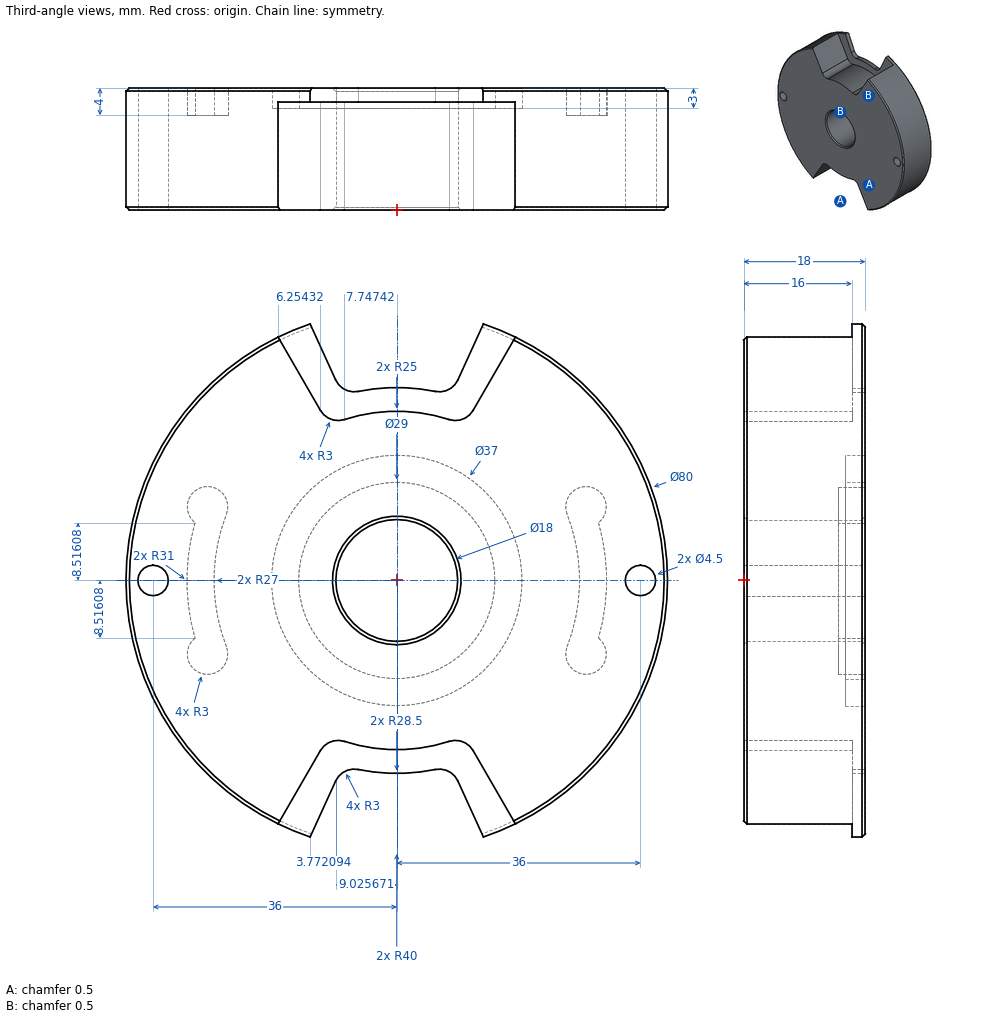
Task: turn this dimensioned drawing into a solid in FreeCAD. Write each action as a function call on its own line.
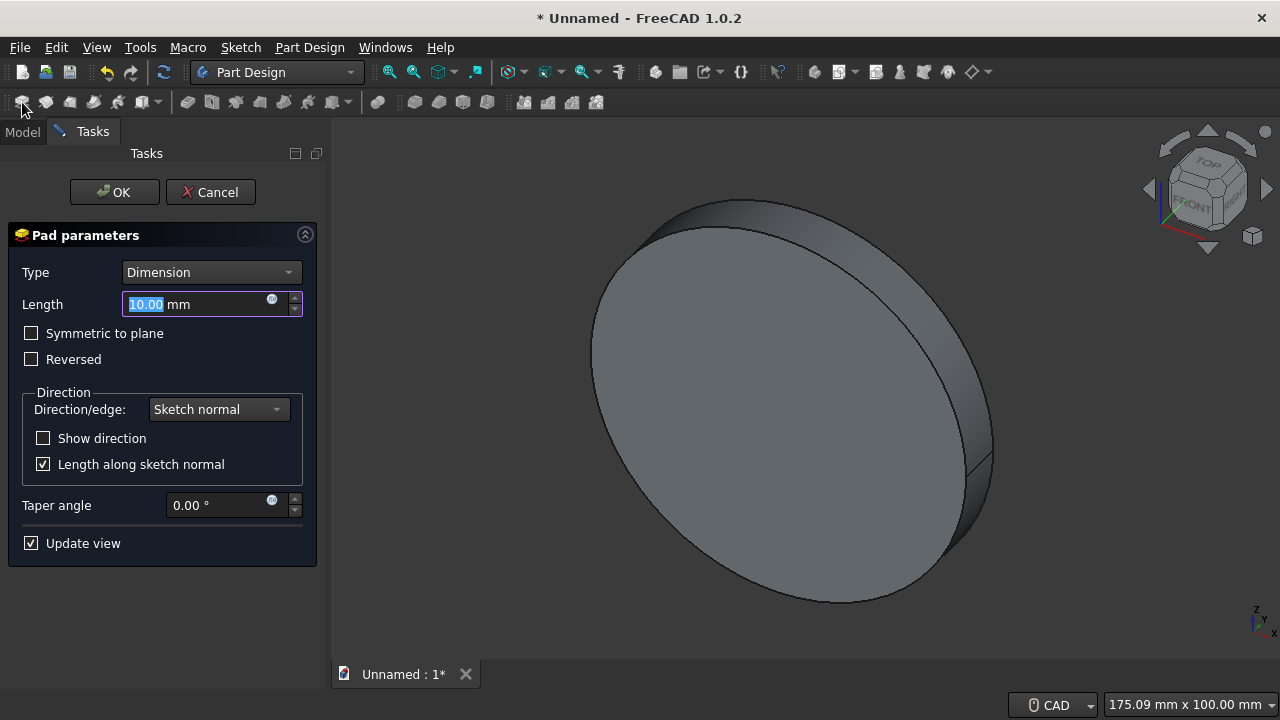
text(18)
key(Tab)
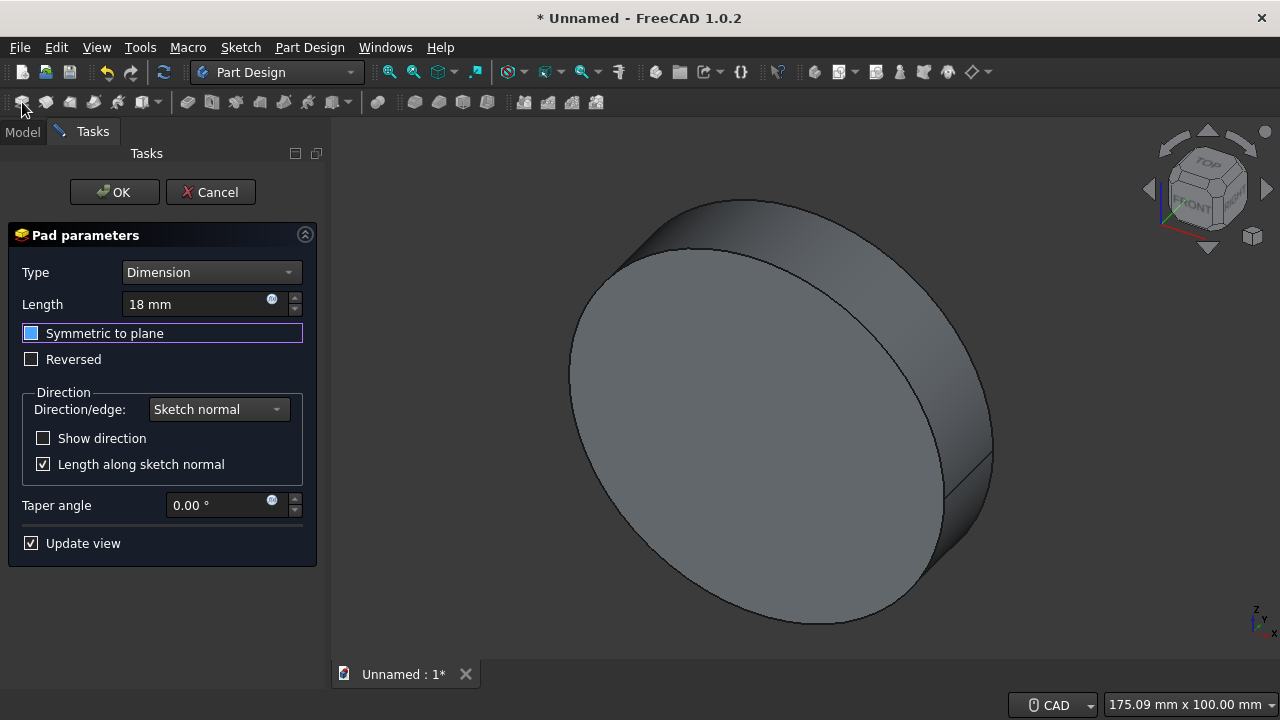
click(30, 359)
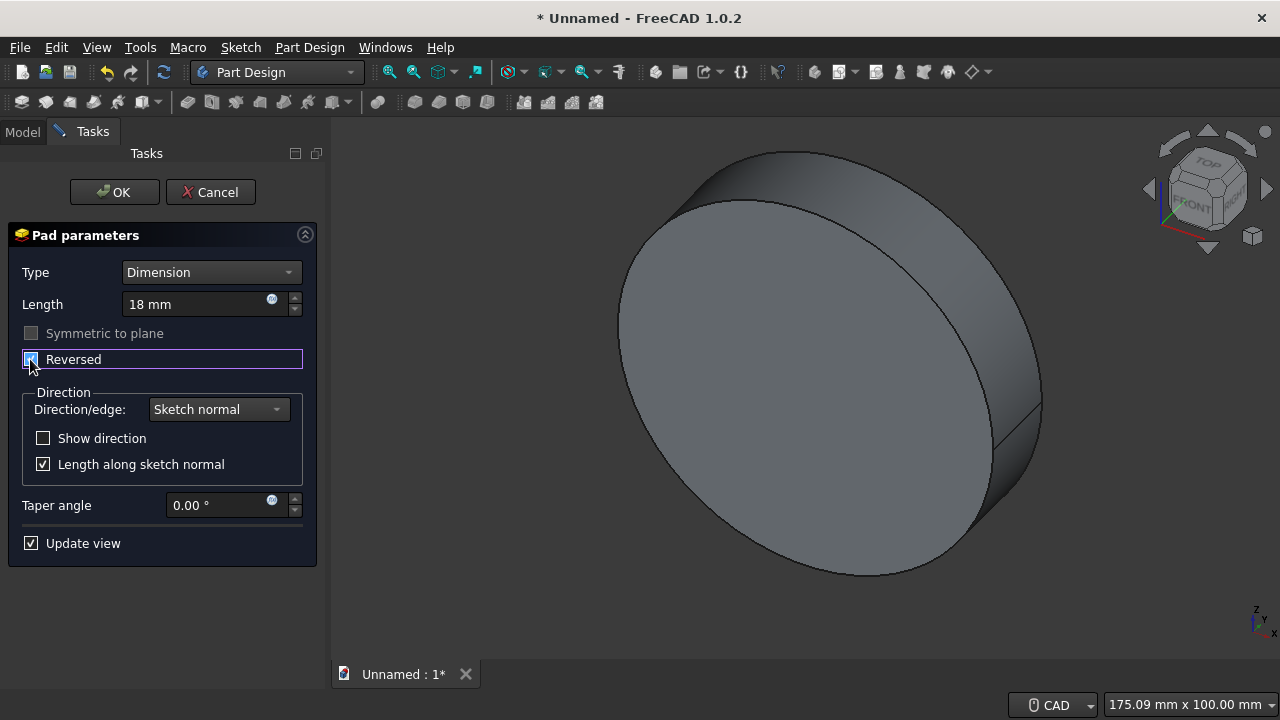
click(115, 192)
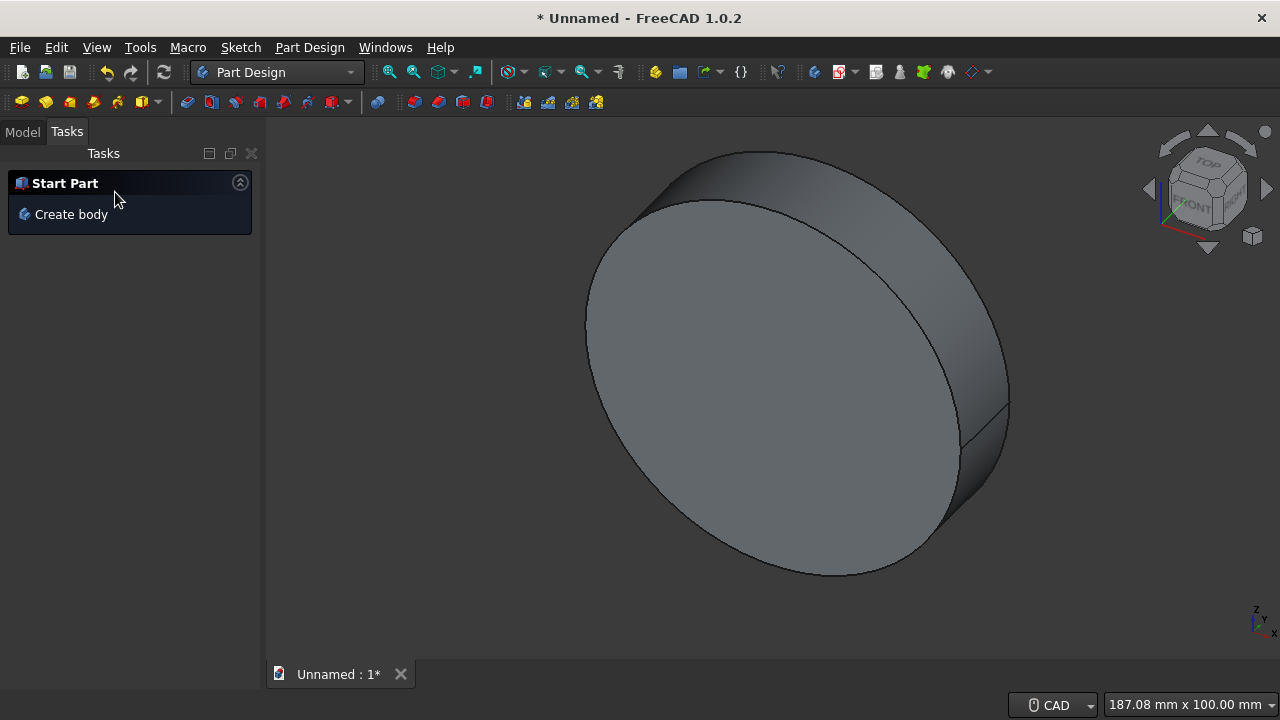
click(390, 72)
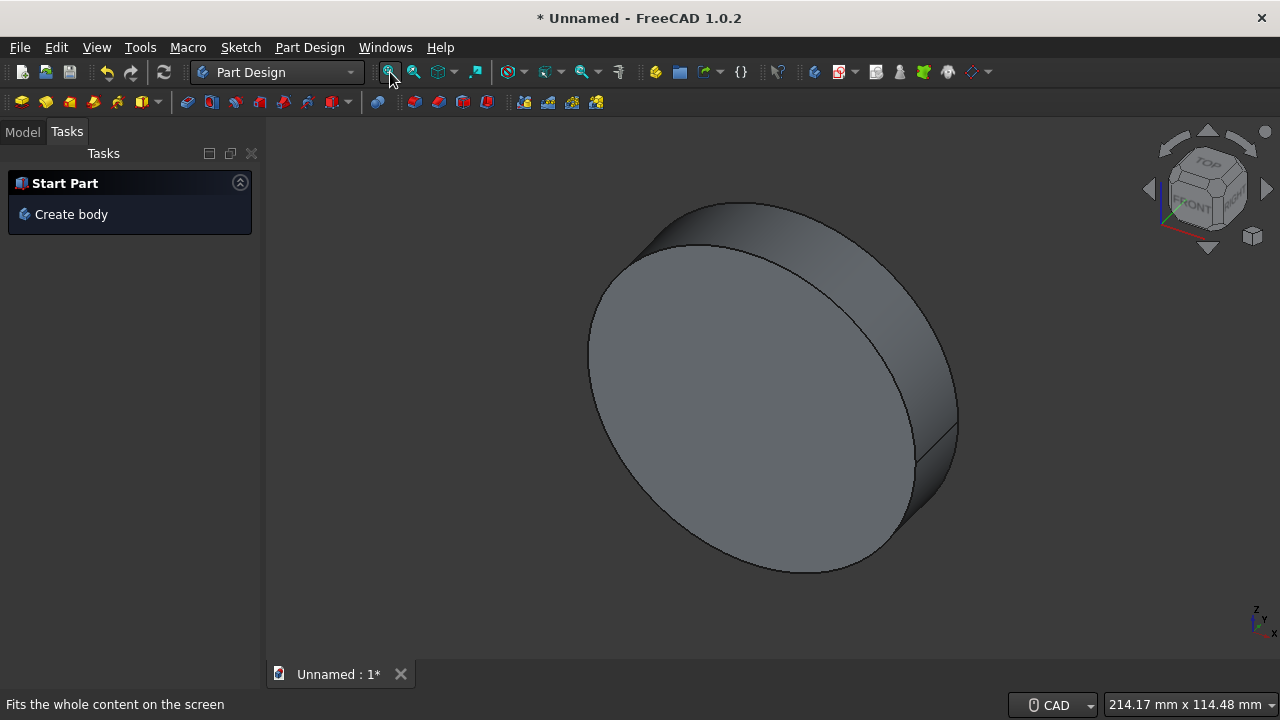
click(619, 273)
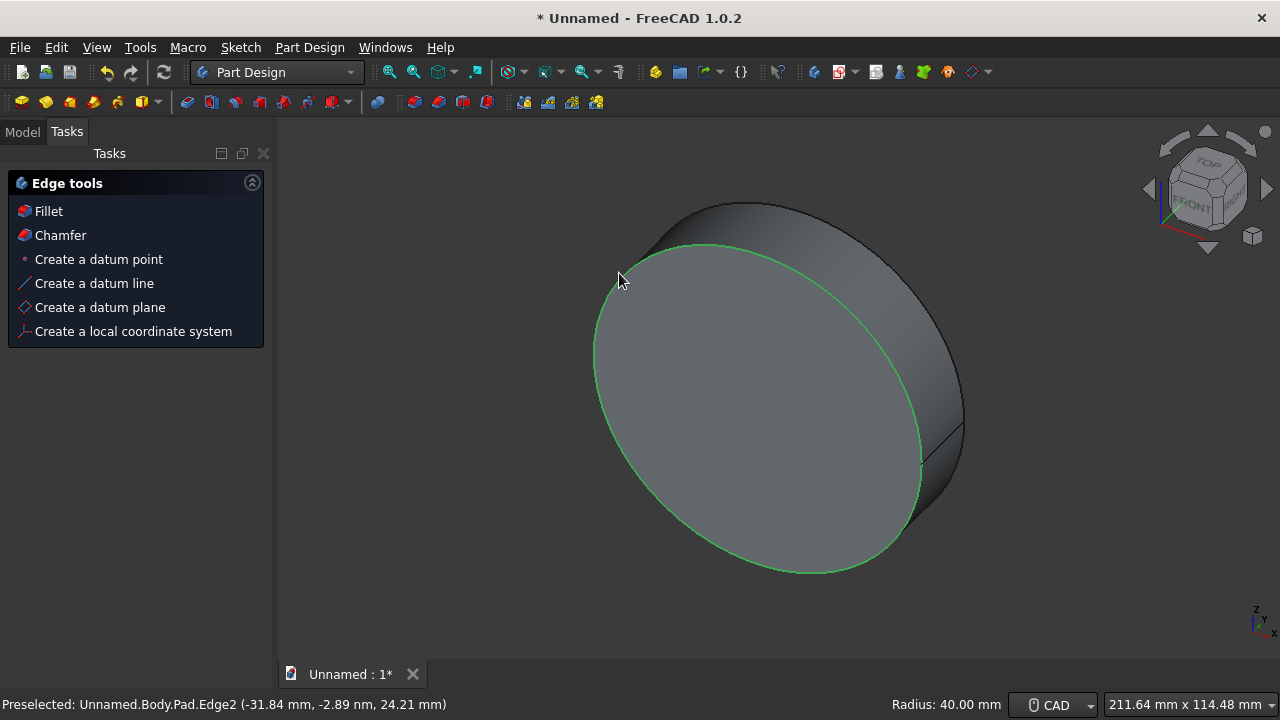
key(0)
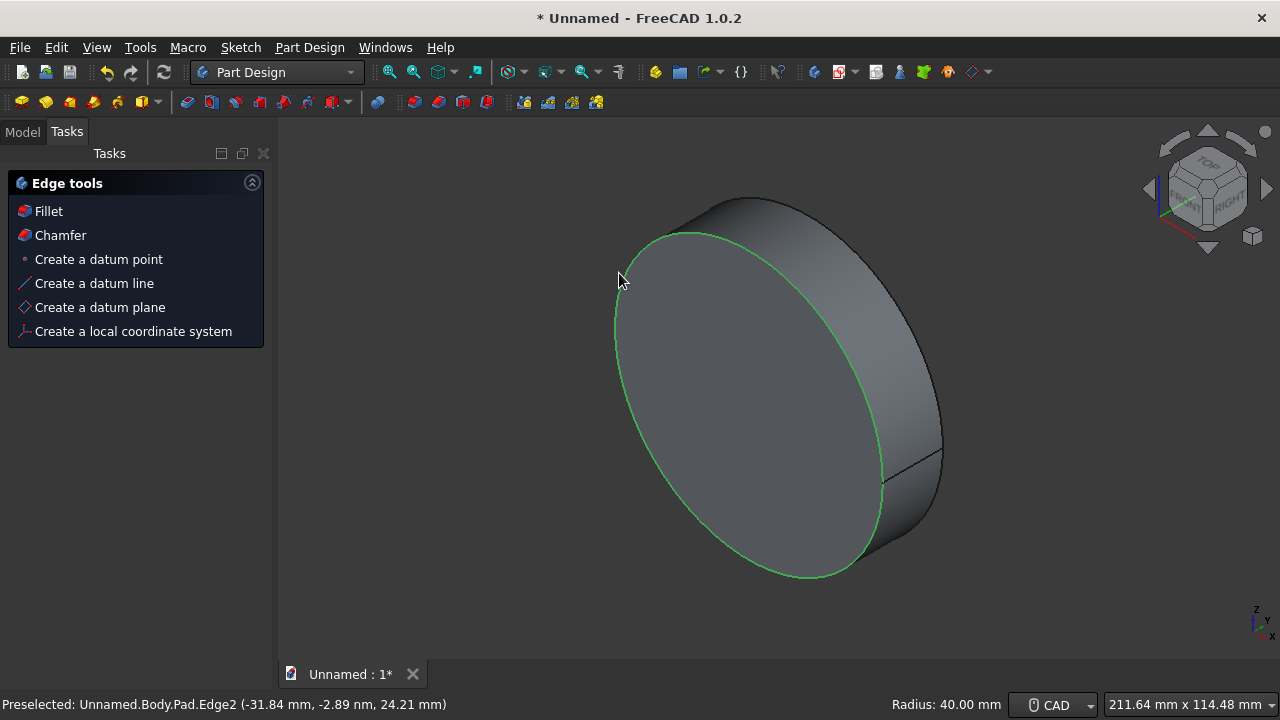
key(2)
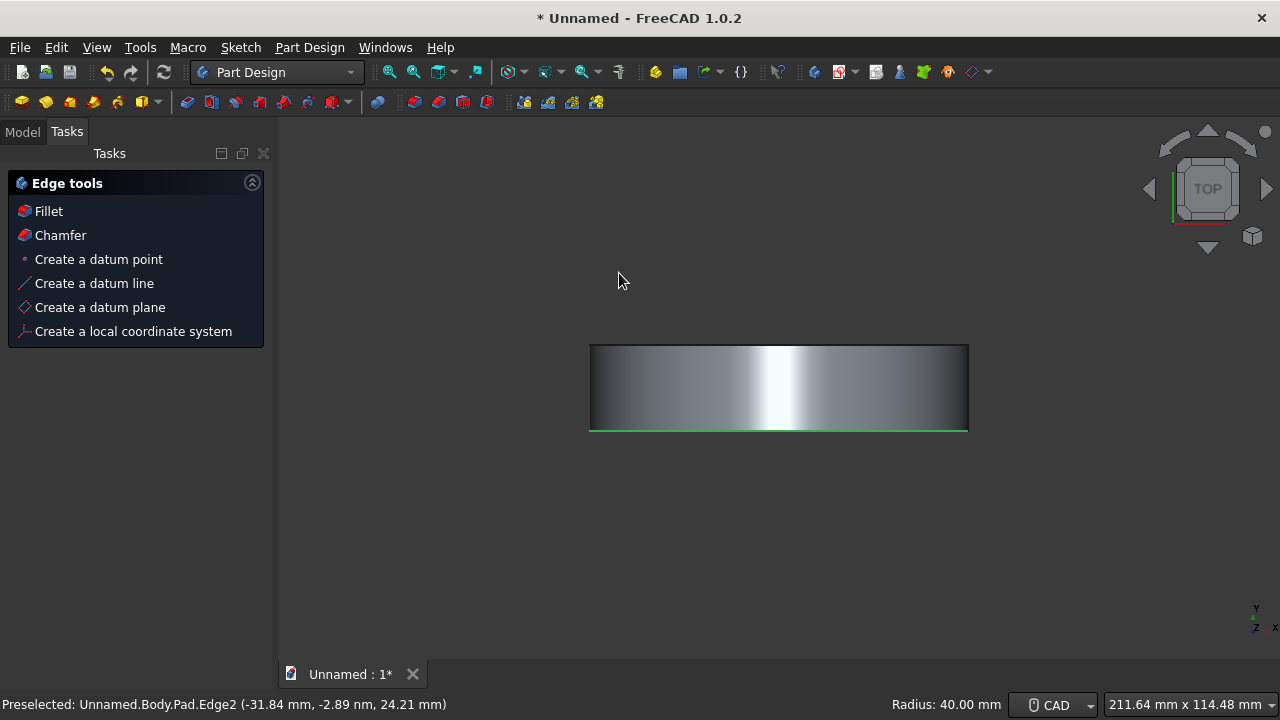
click(390, 72)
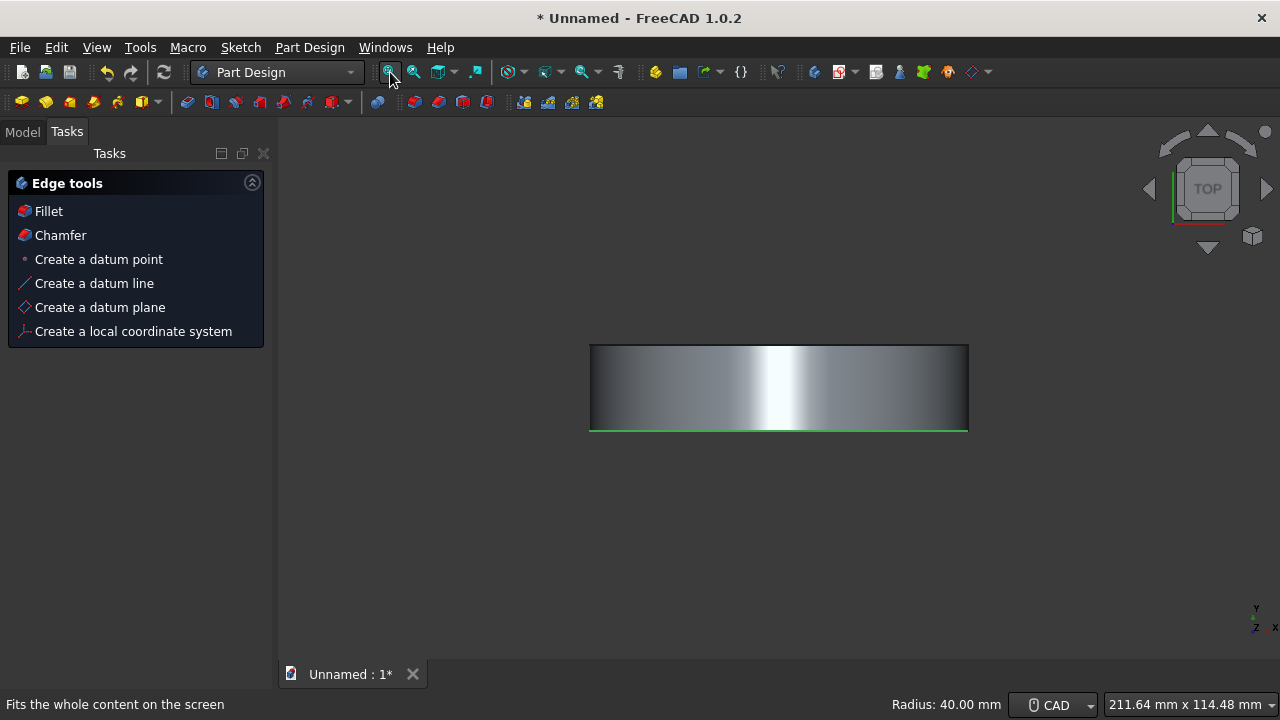
click(626, 344, ctrl)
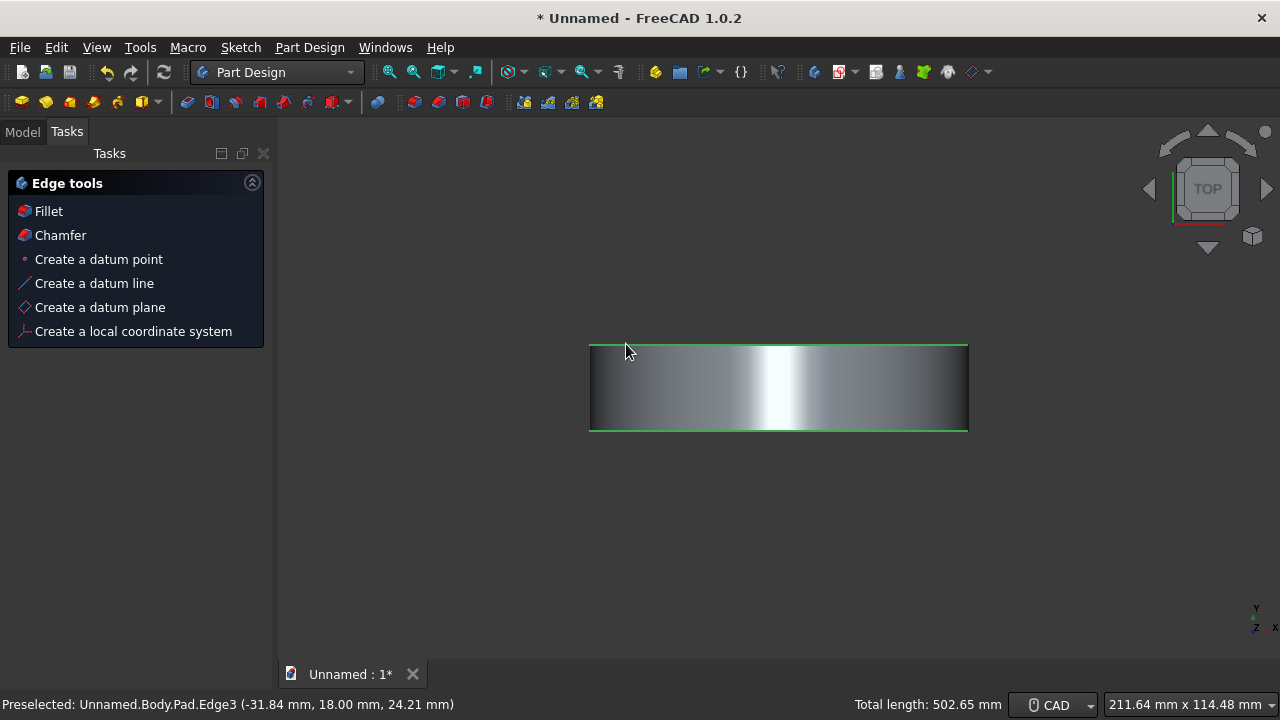
click(440, 102)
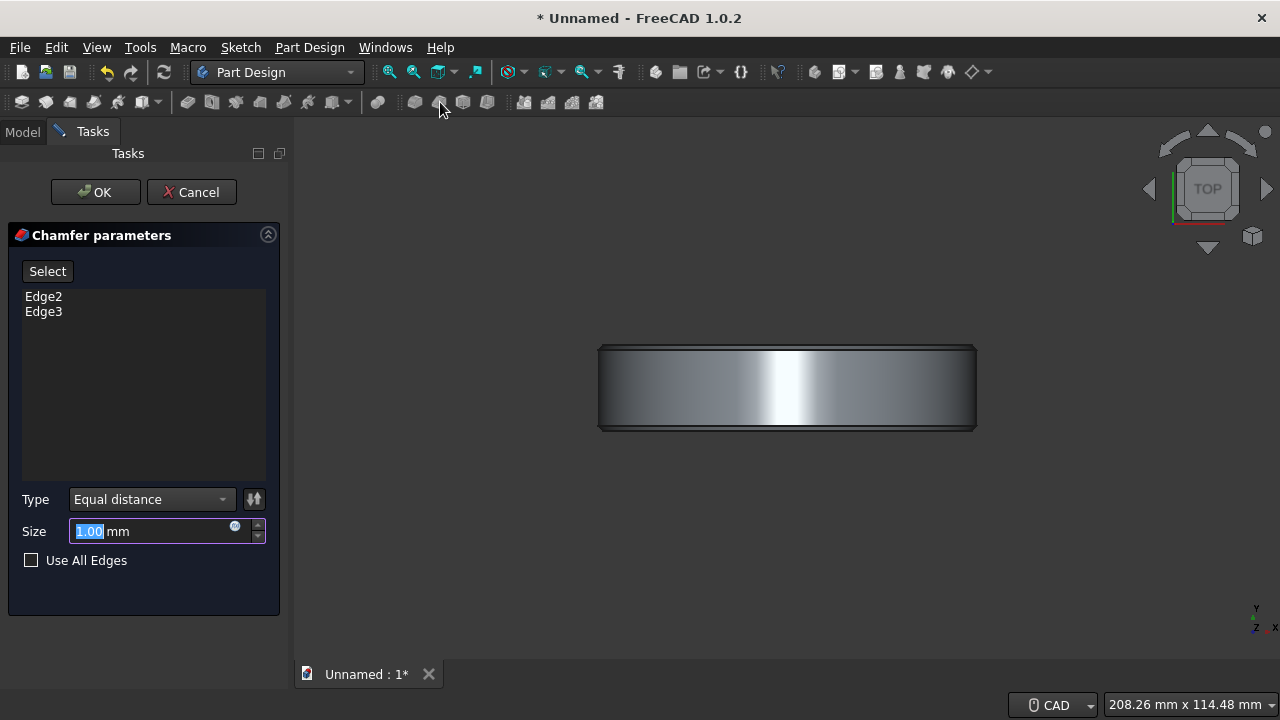
text(0.5)
key(Tab)